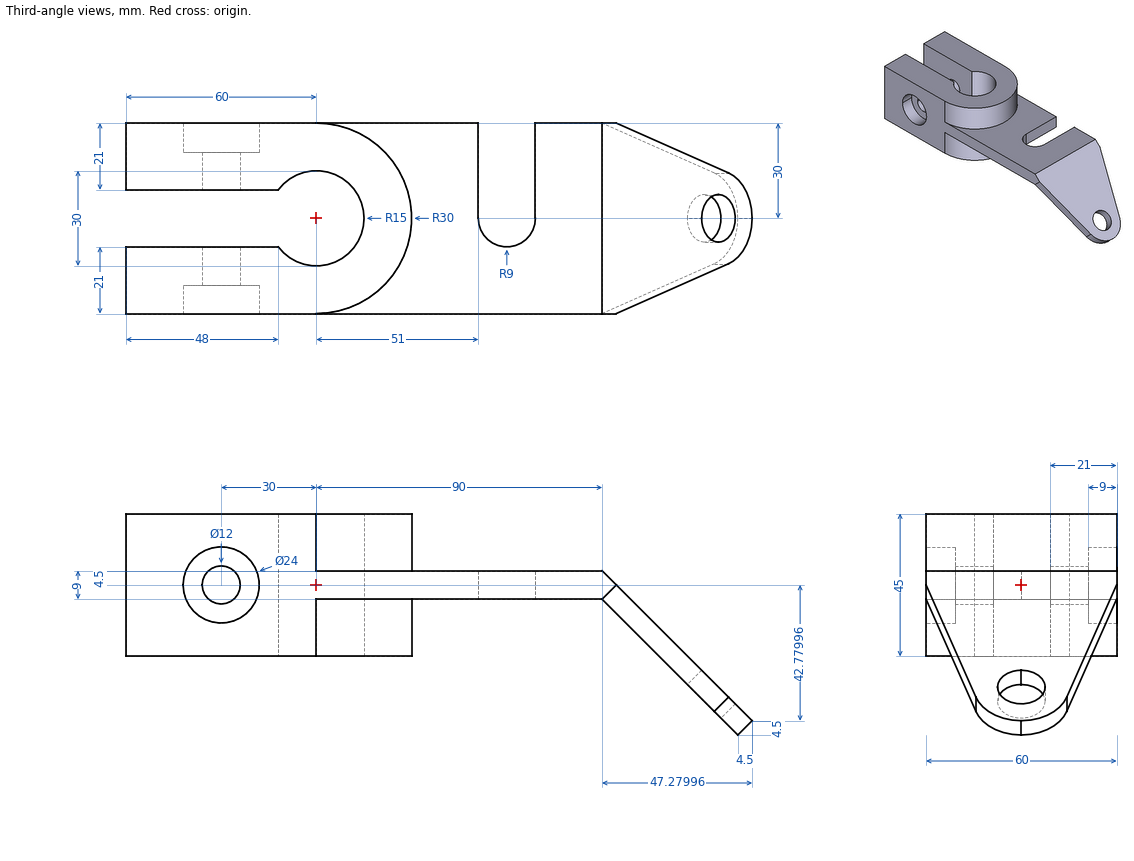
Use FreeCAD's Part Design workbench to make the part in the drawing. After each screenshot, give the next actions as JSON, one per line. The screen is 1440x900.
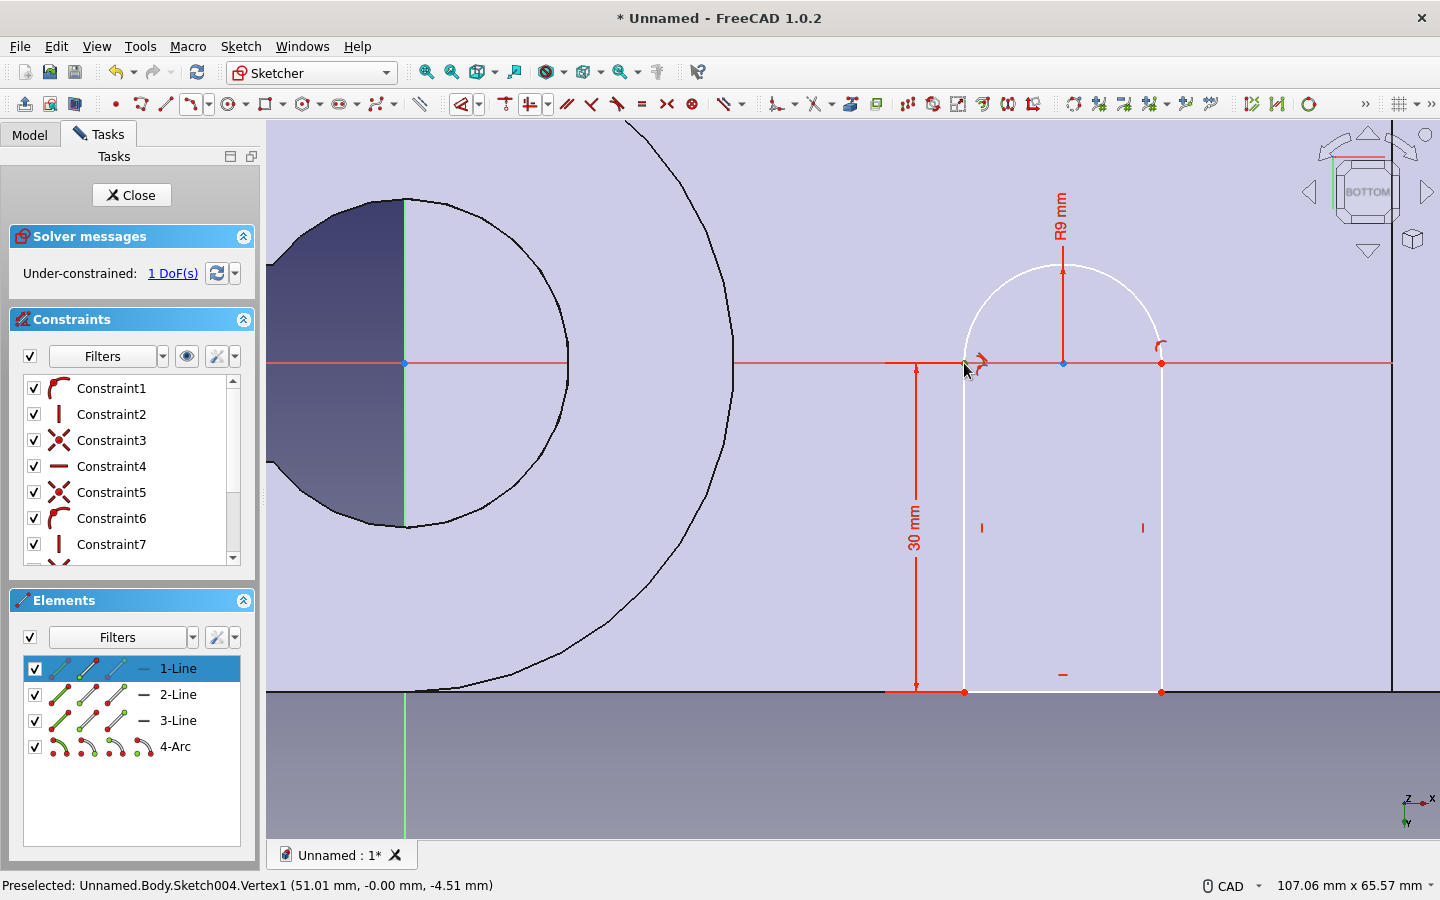
{"action": "key", "text": "l"}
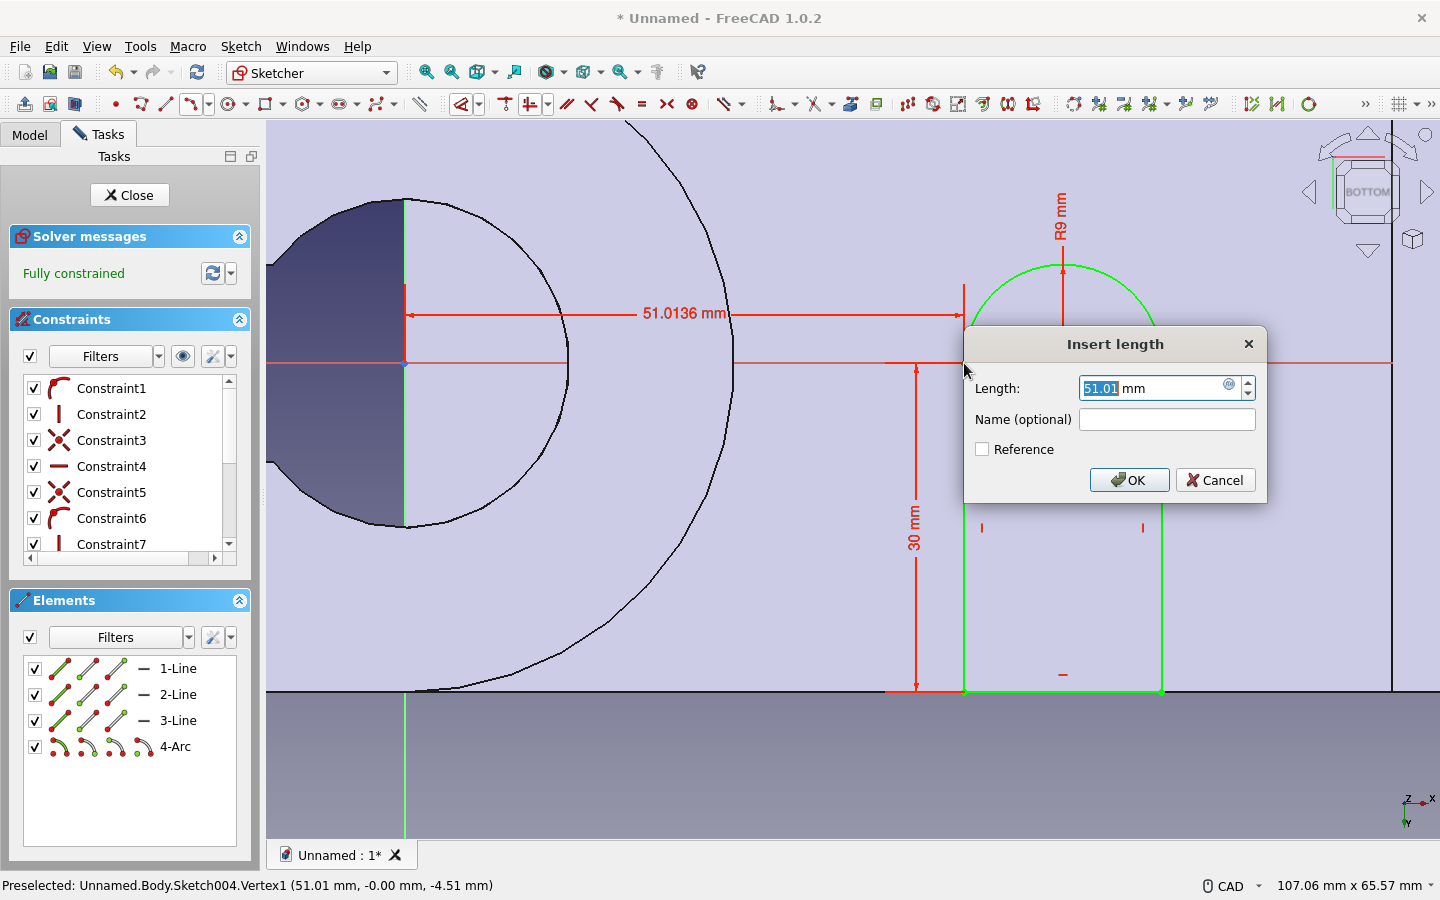
{"action": "type", "text": "51"}
{"action": "key", "text": "Return"}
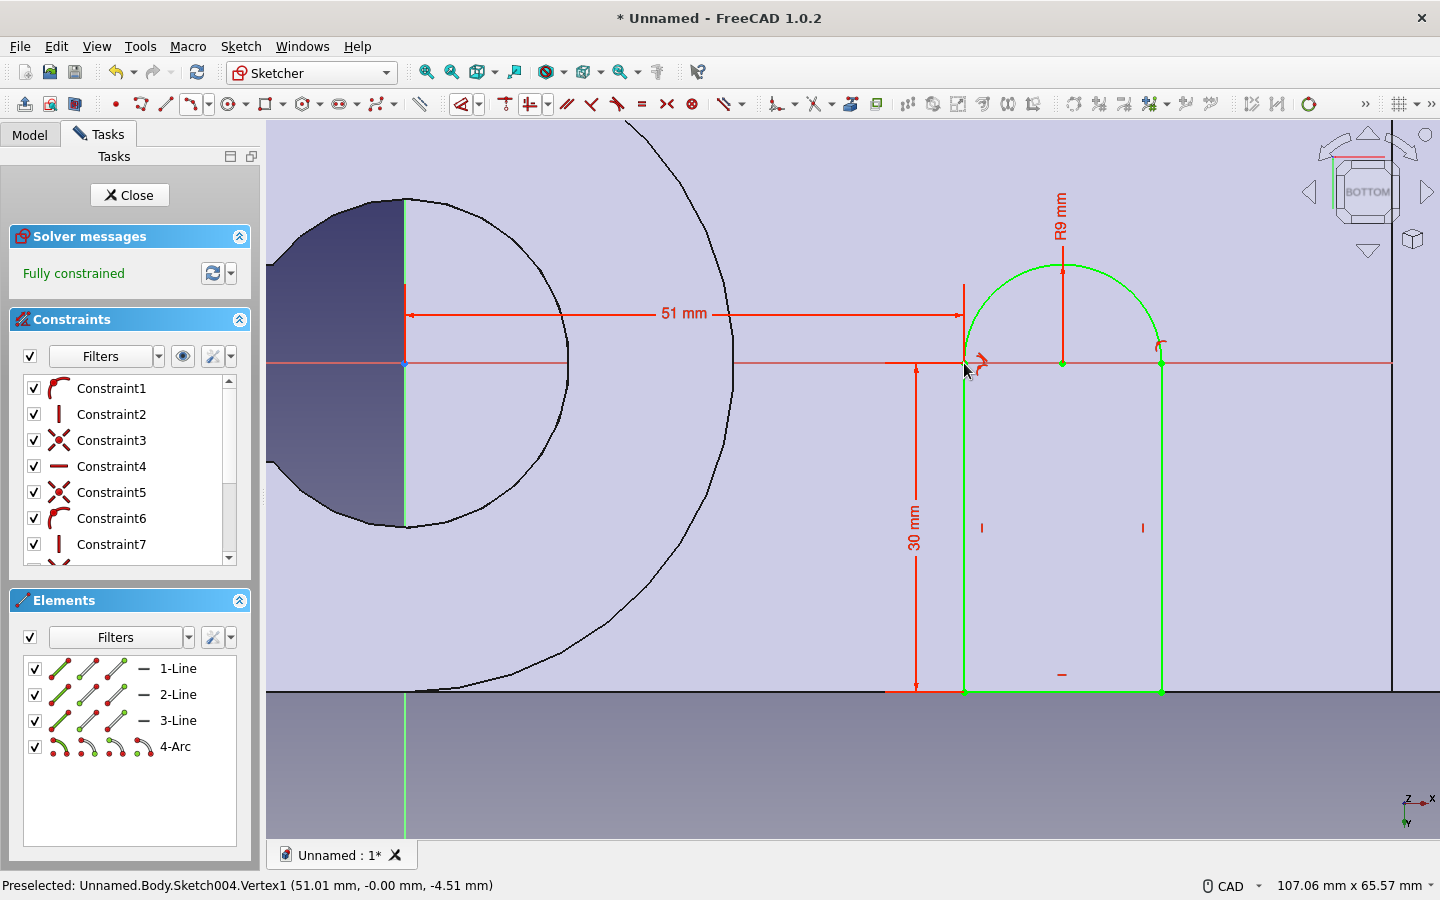
{"action": "left_click", "coordinate": [130, 195]}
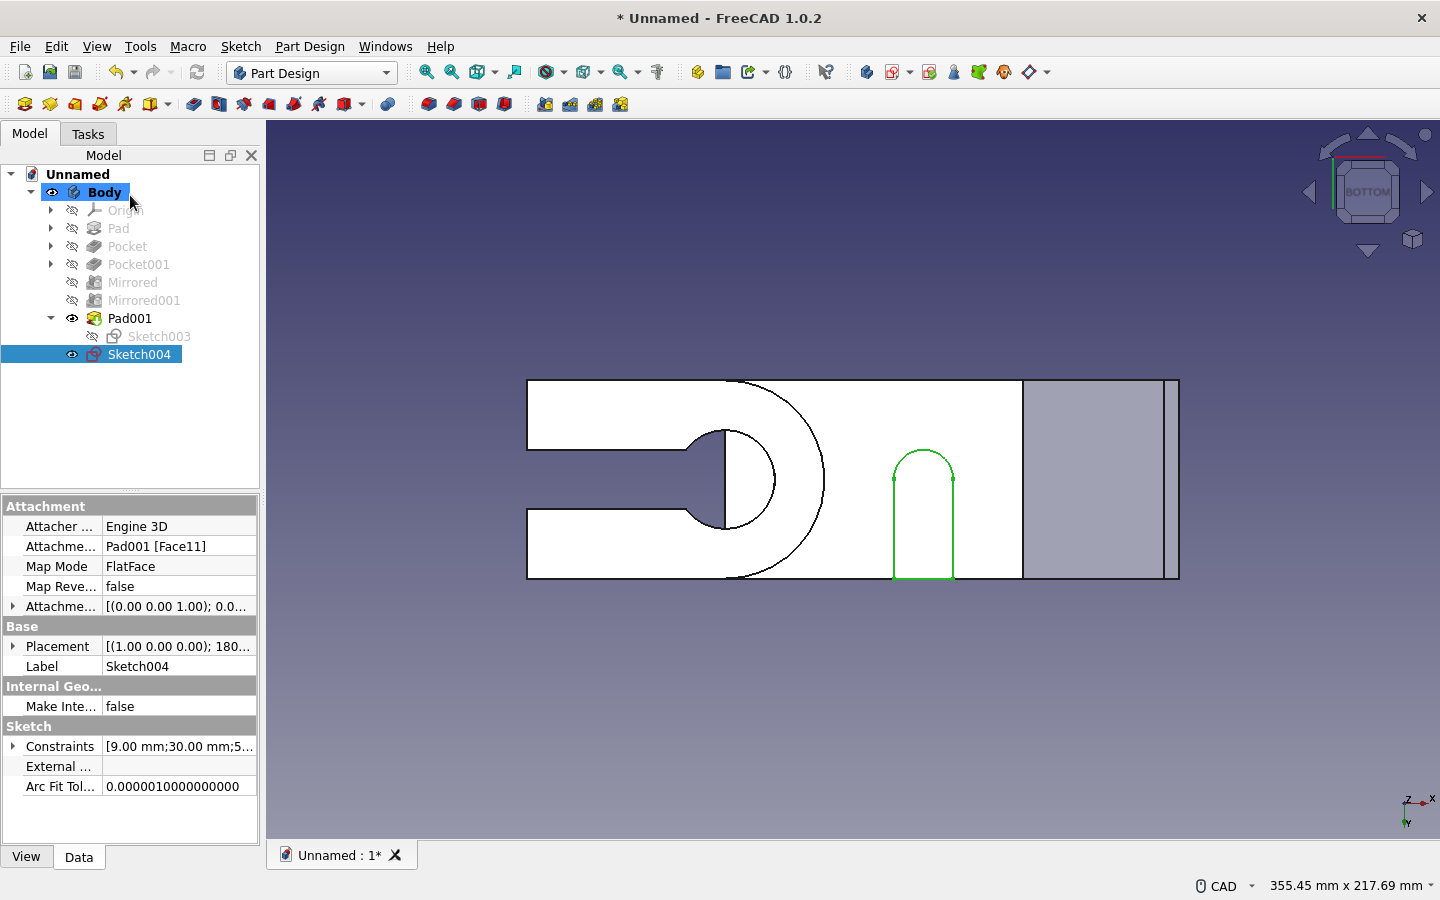
{"action": "left_click", "coordinate": [194, 104]}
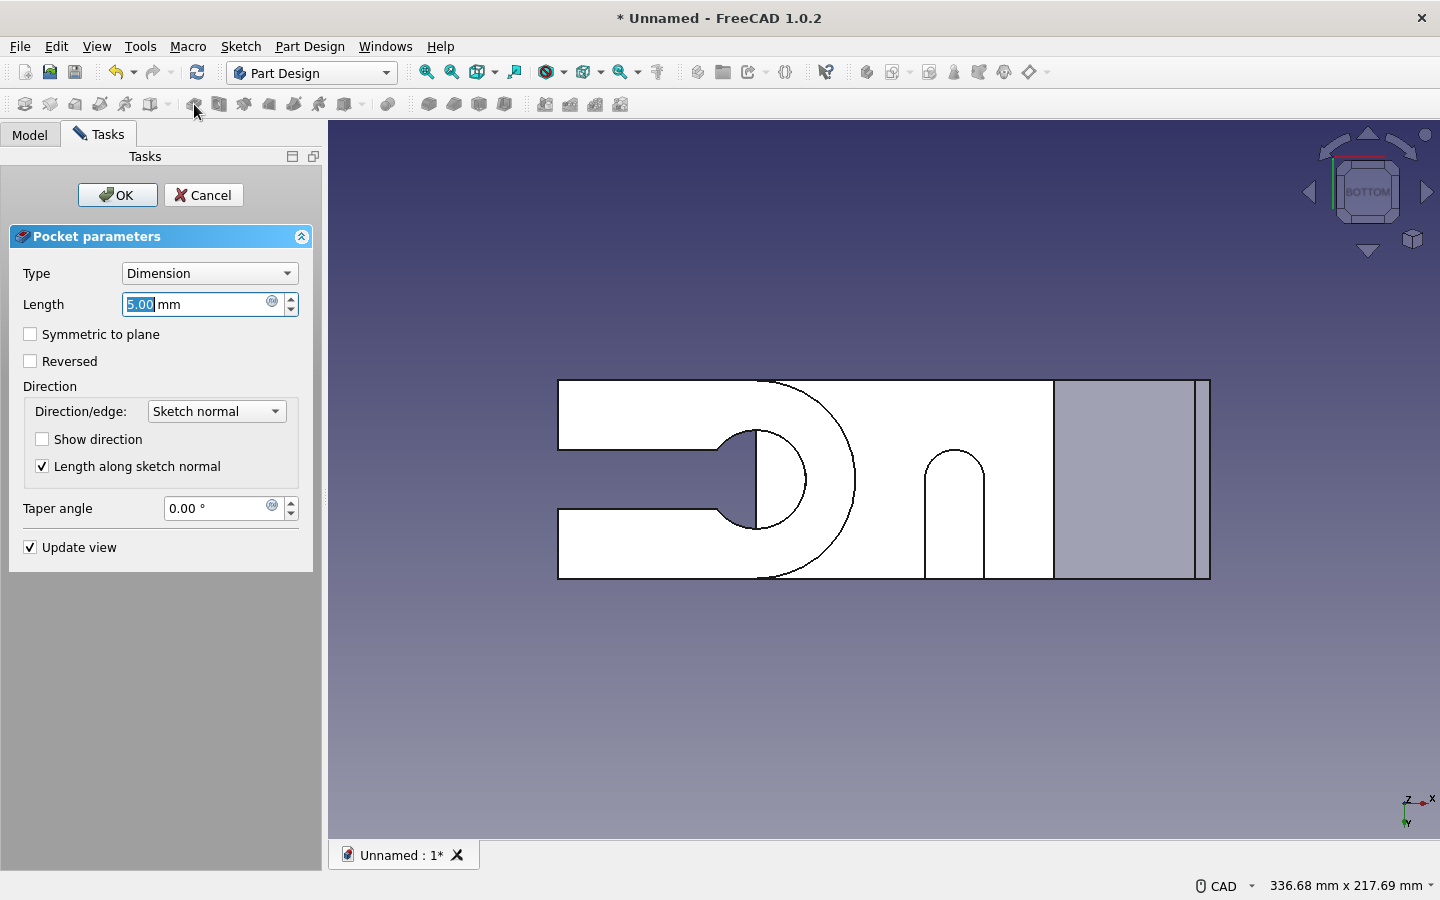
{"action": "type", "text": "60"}
{"action": "key", "text": "Tab"}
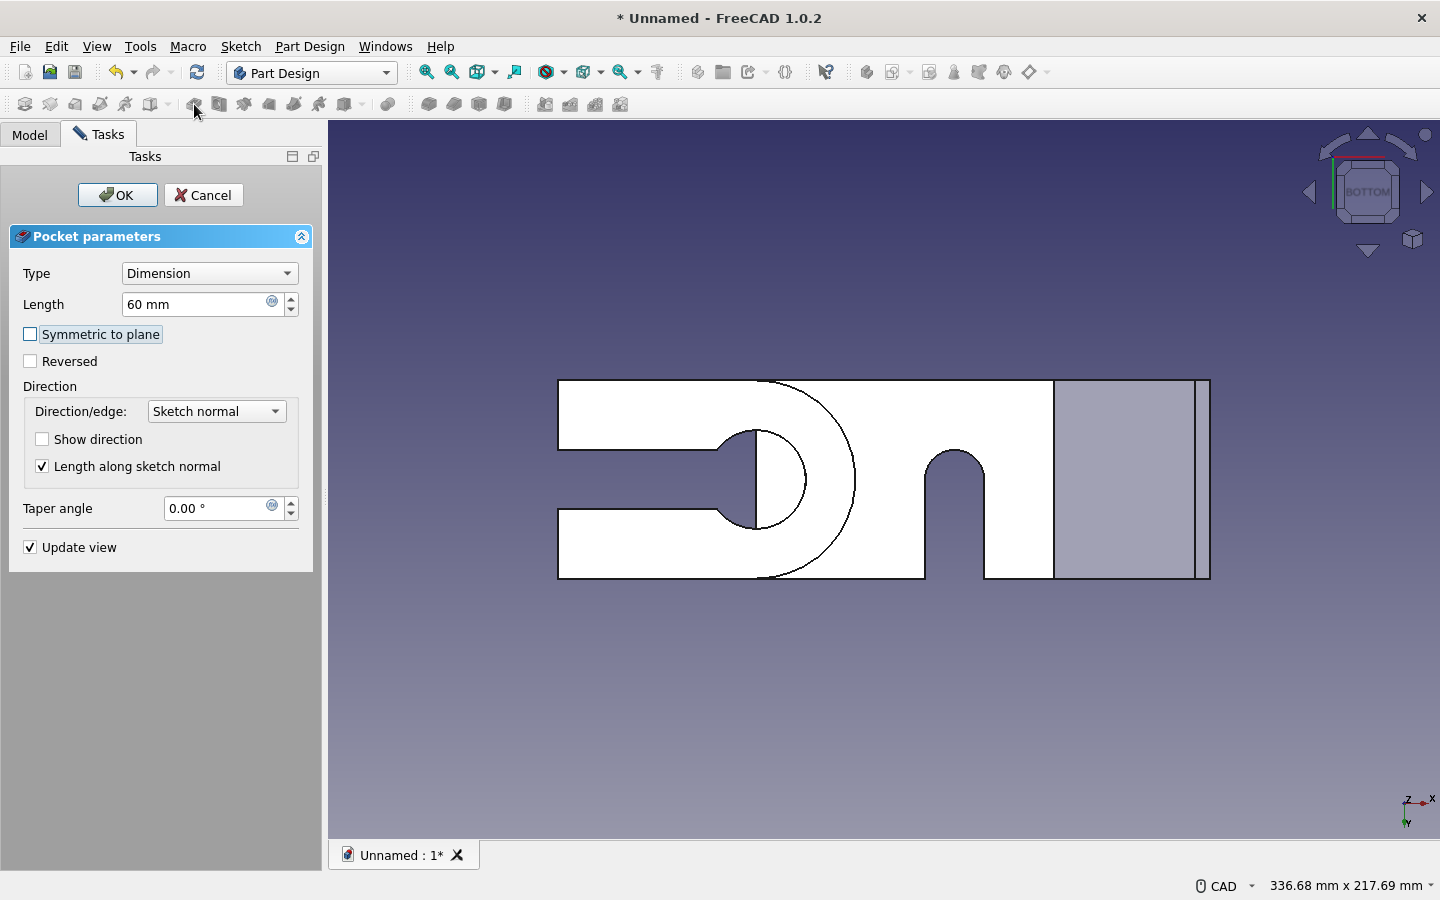
{"action": "left_click", "coordinate": [31, 334]}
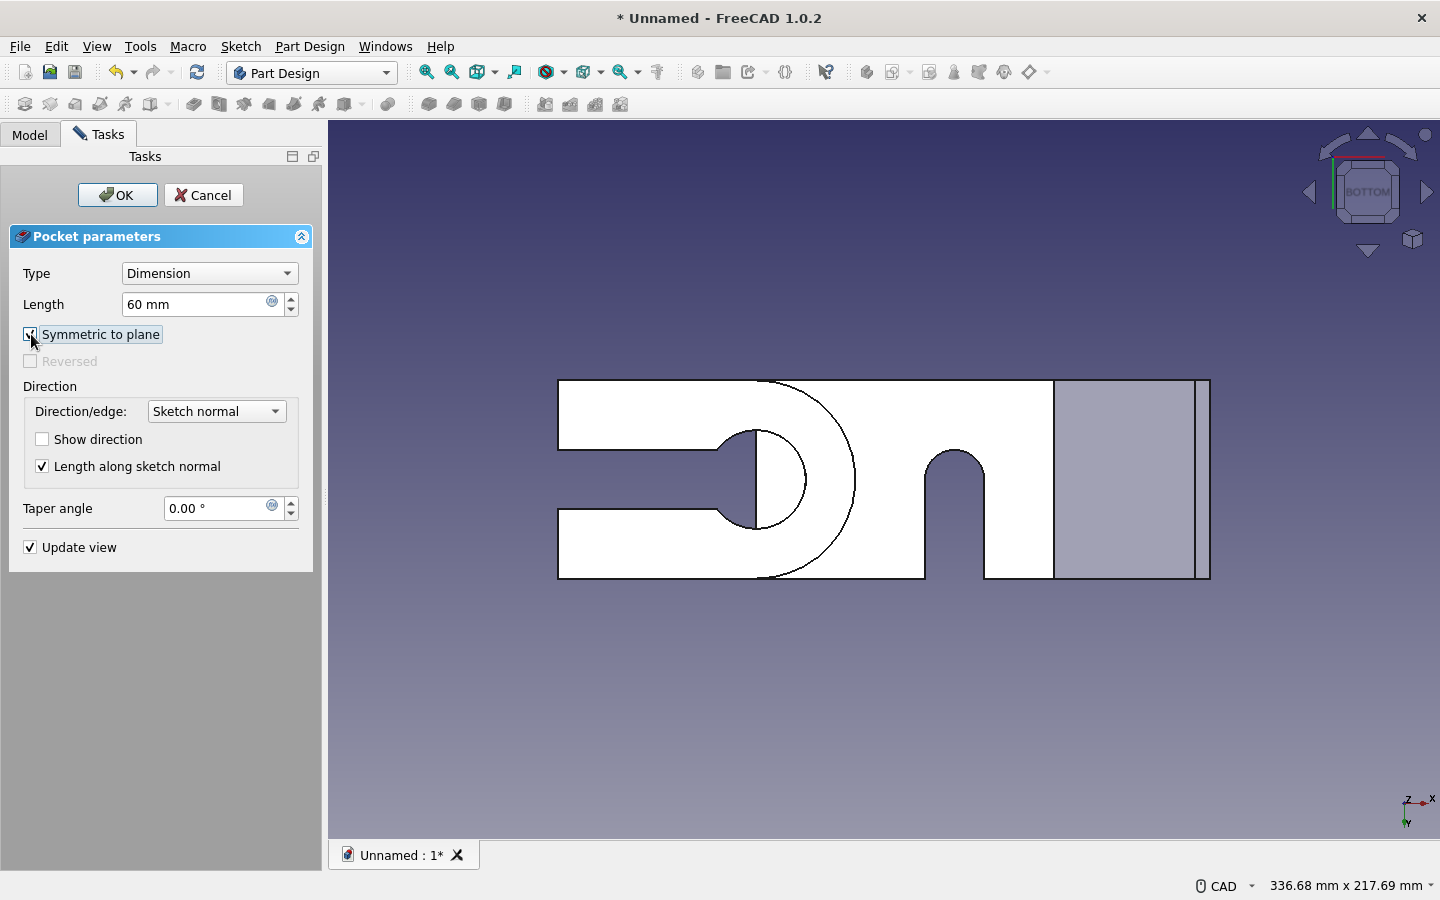
{"action": "left_click", "coordinate": [118, 195]}